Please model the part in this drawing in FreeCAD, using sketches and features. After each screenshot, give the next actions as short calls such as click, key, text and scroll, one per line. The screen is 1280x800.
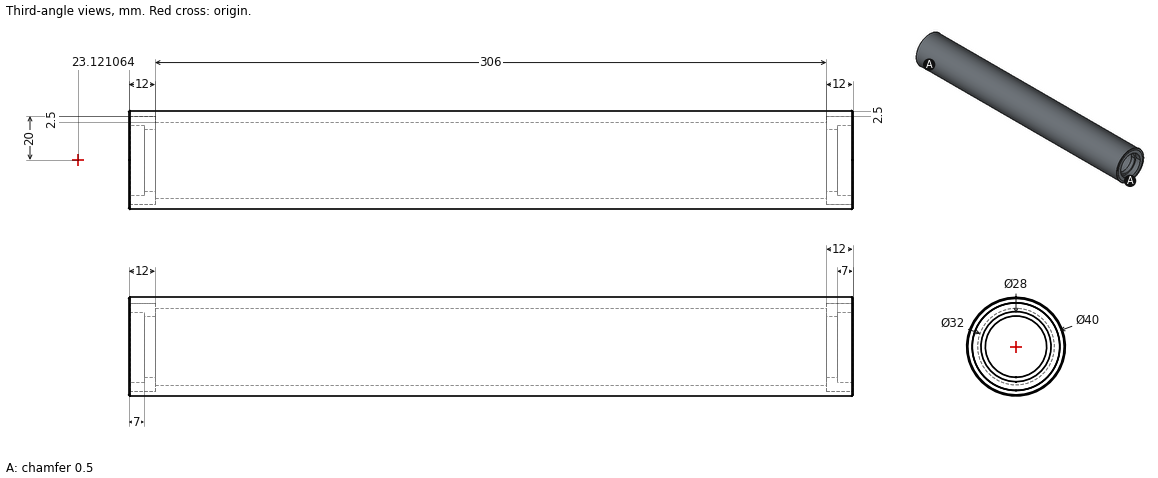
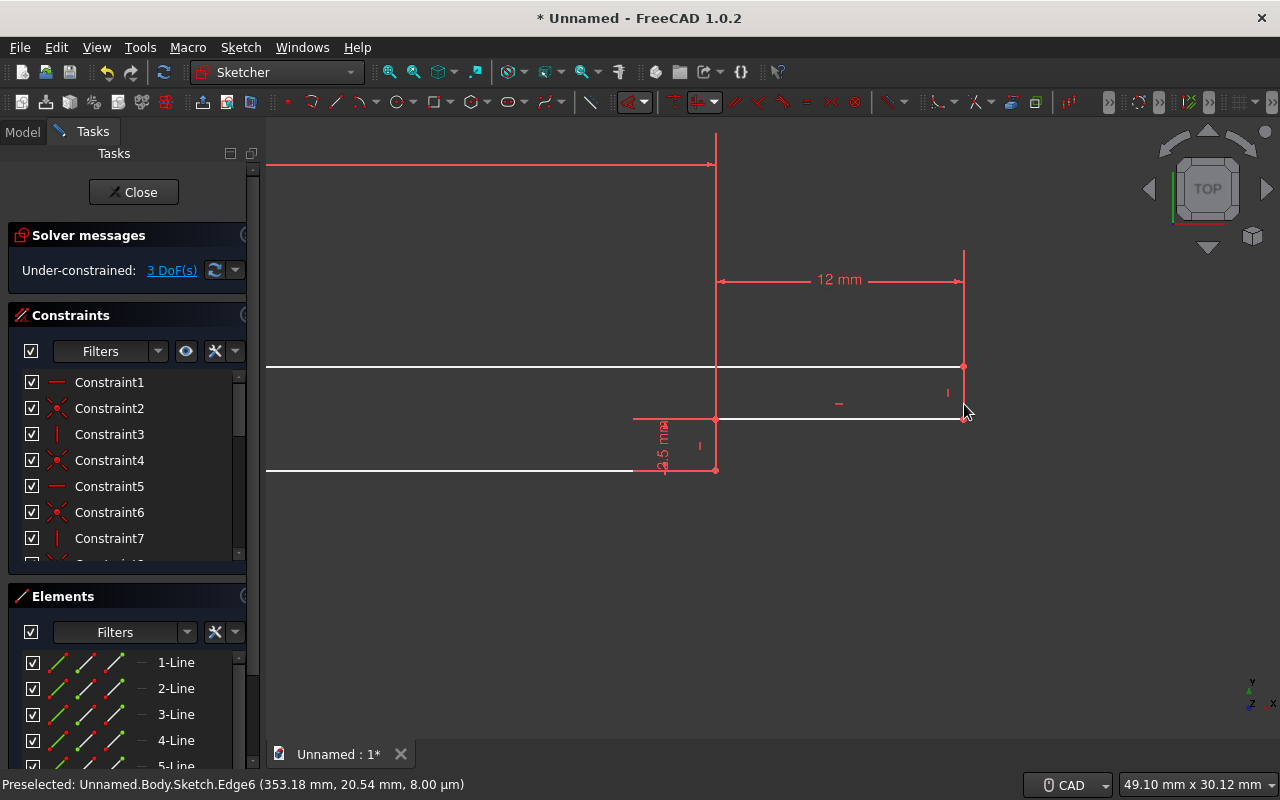
key(i)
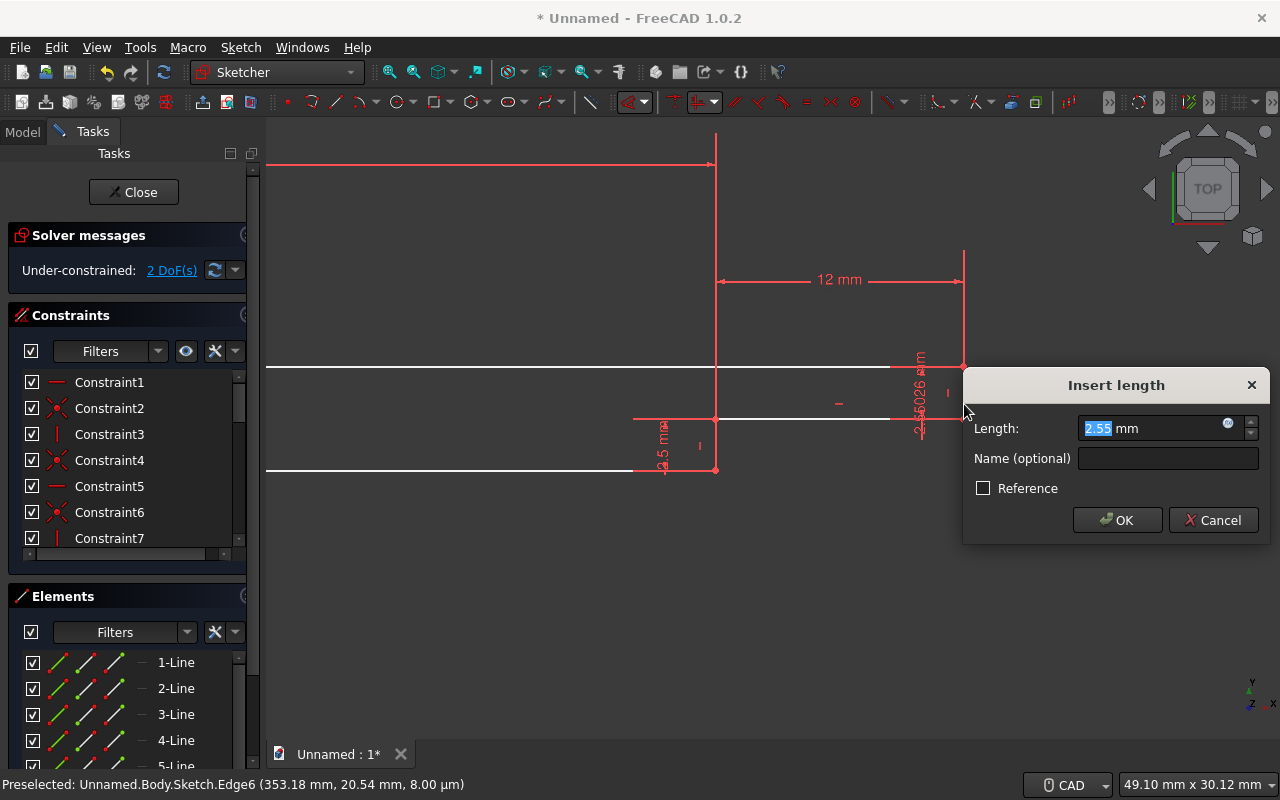
text(2.5)
key(Return)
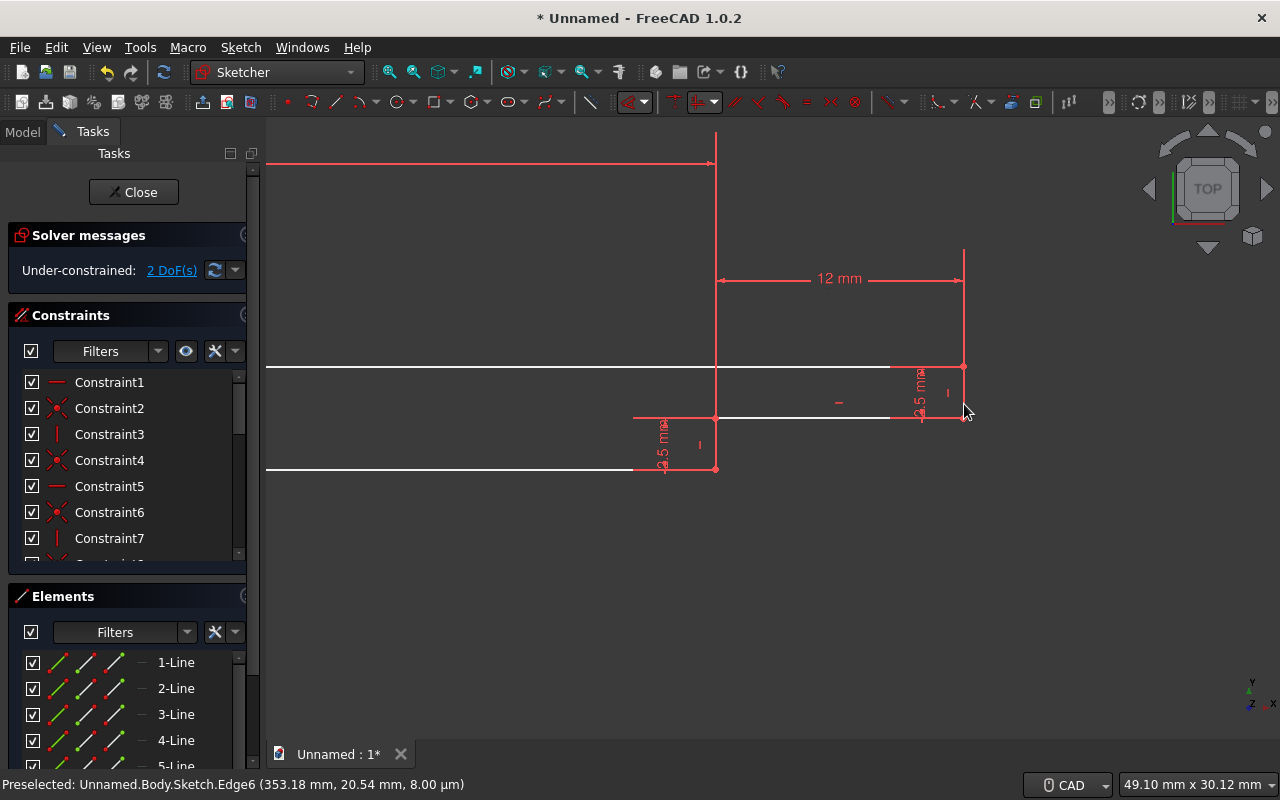
scroll(976, 414, down, 13)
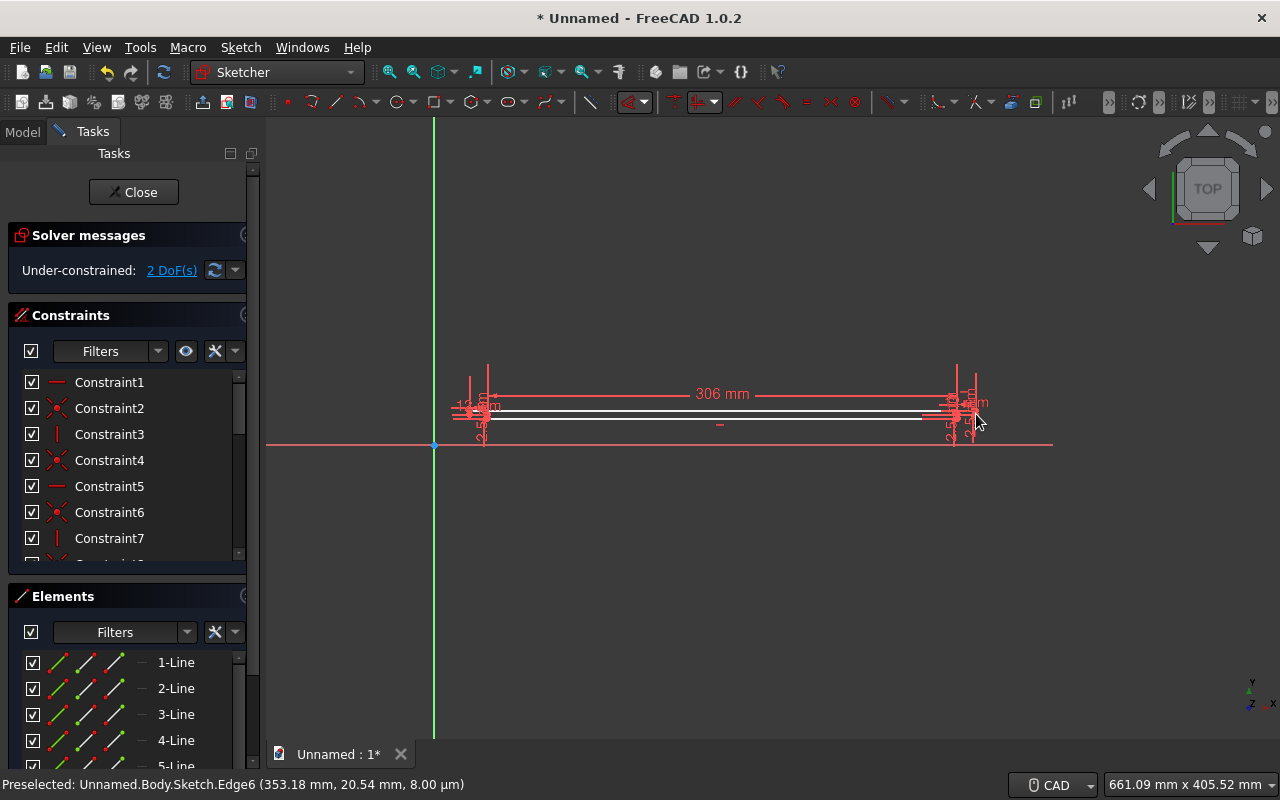
scroll(470, 415, up, 6)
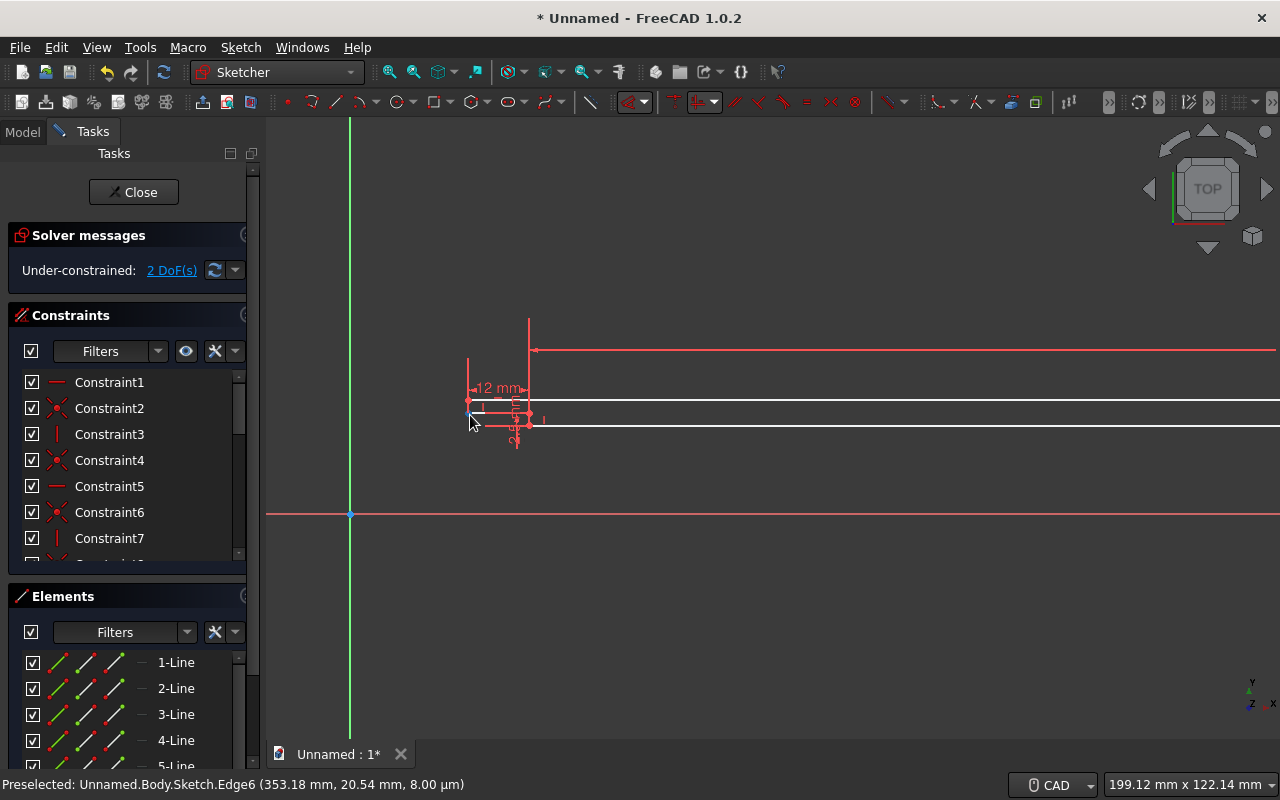
click(468, 413)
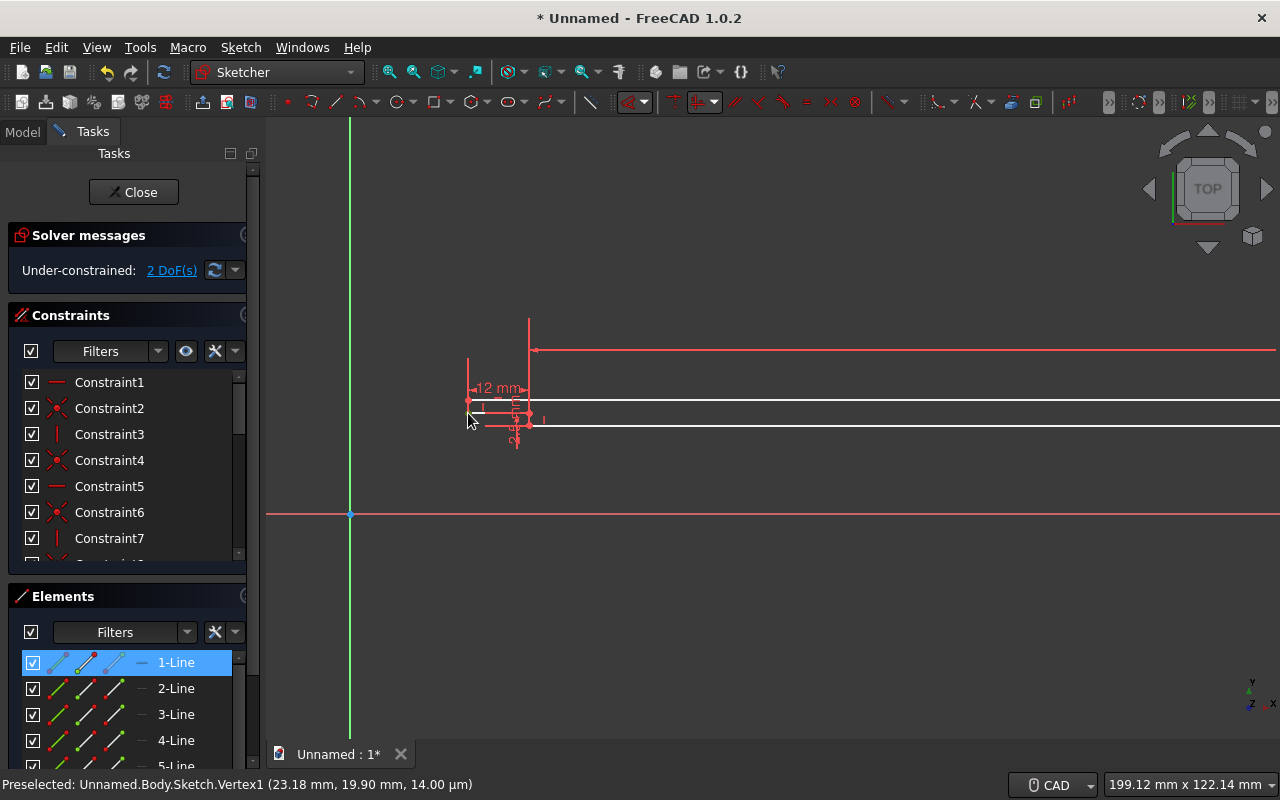
click(646, 102)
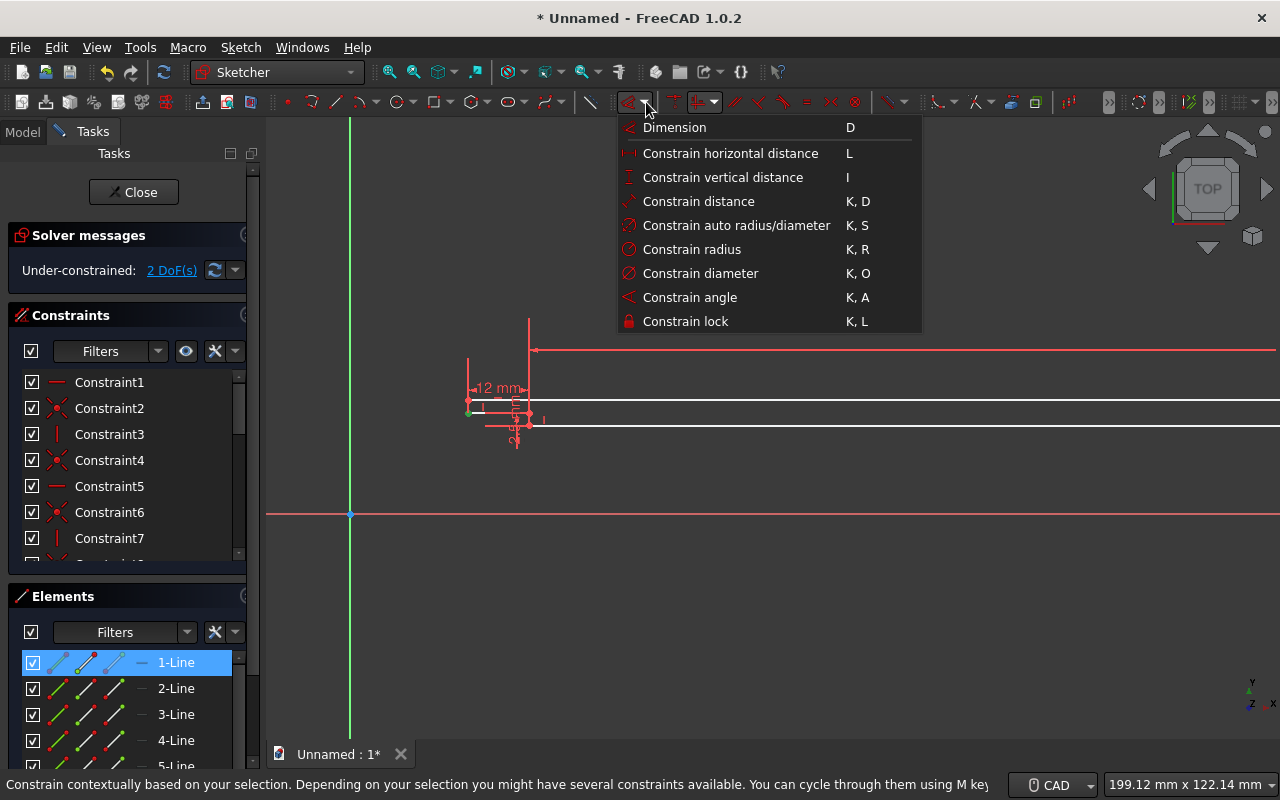
click(770, 177)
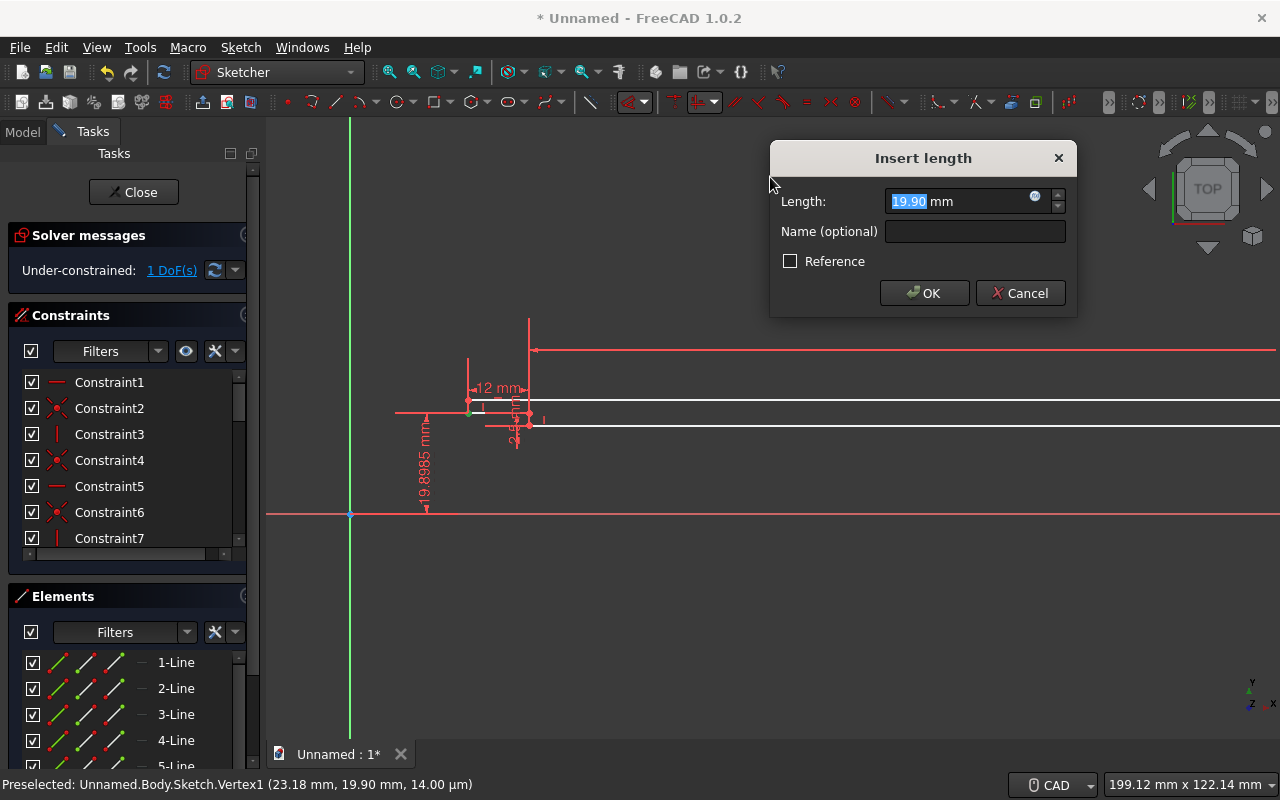
text(20)
key(Return)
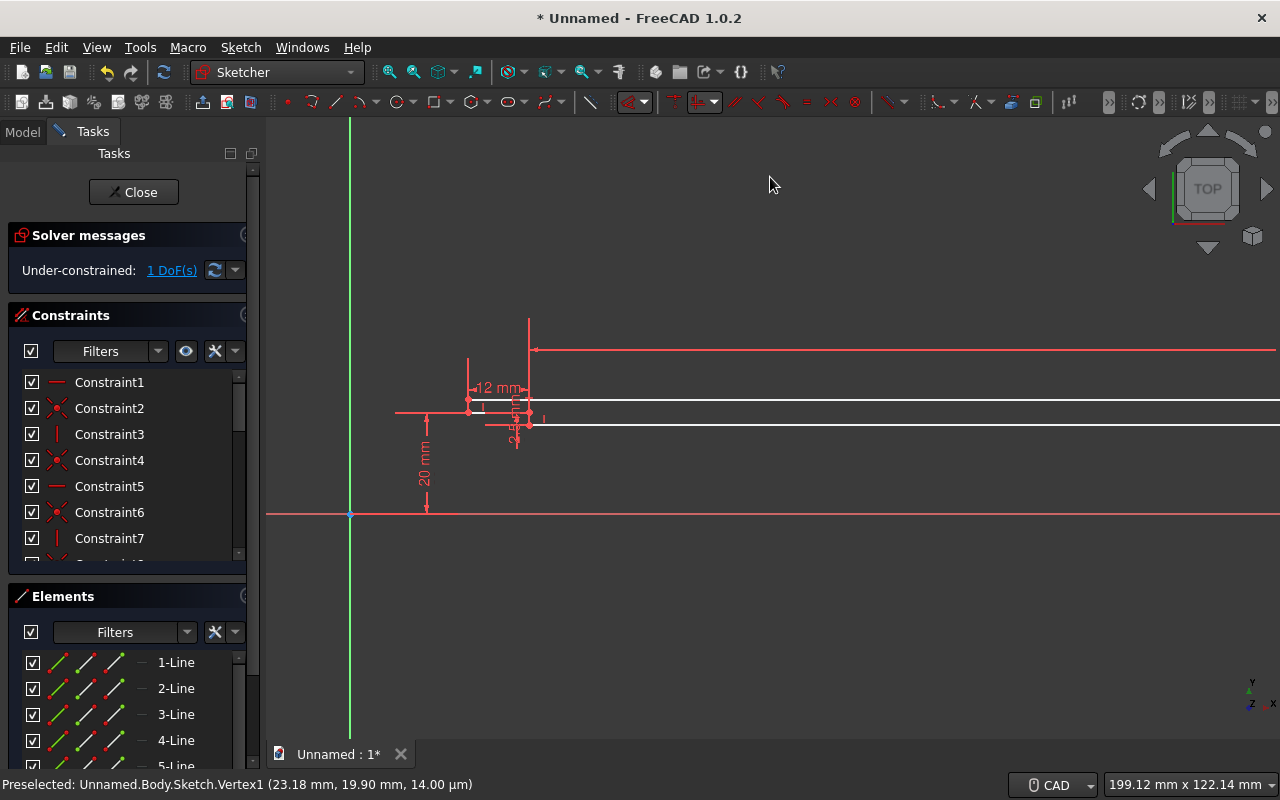
click(468, 413)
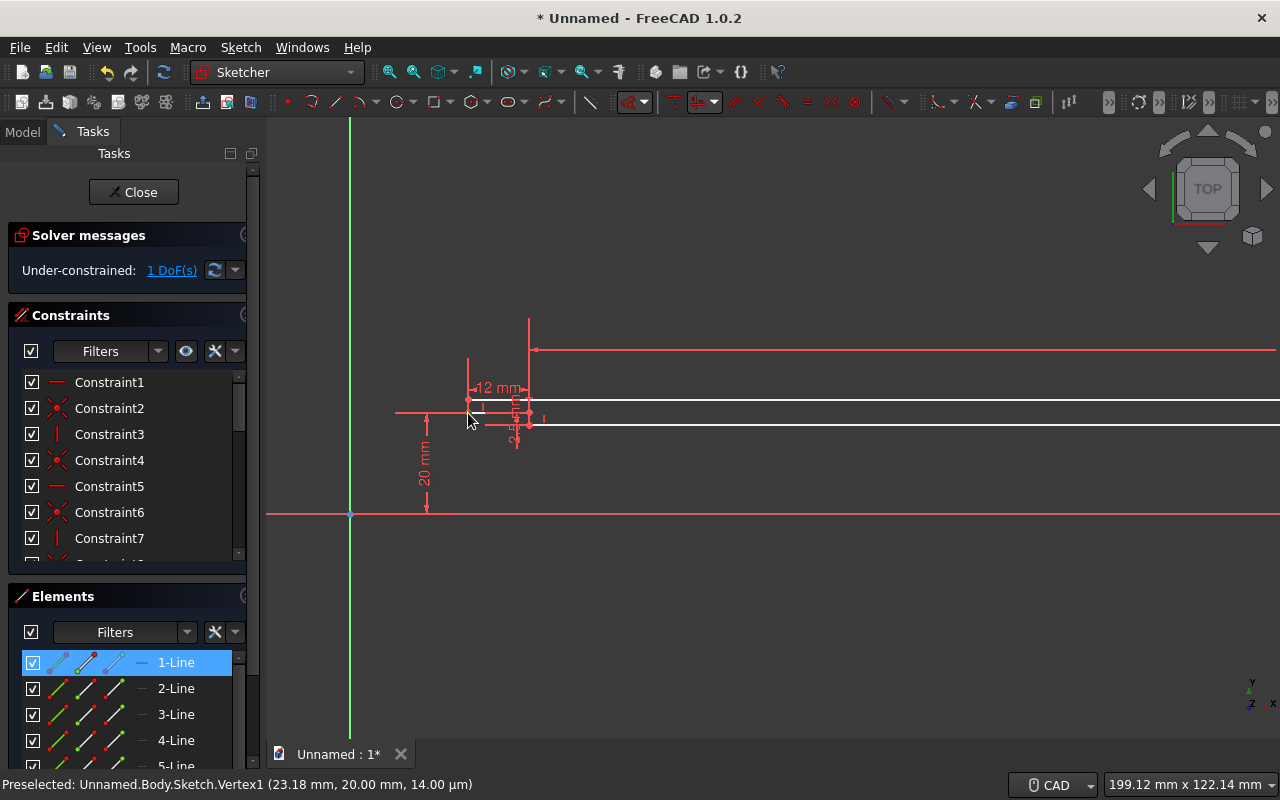
key(l)